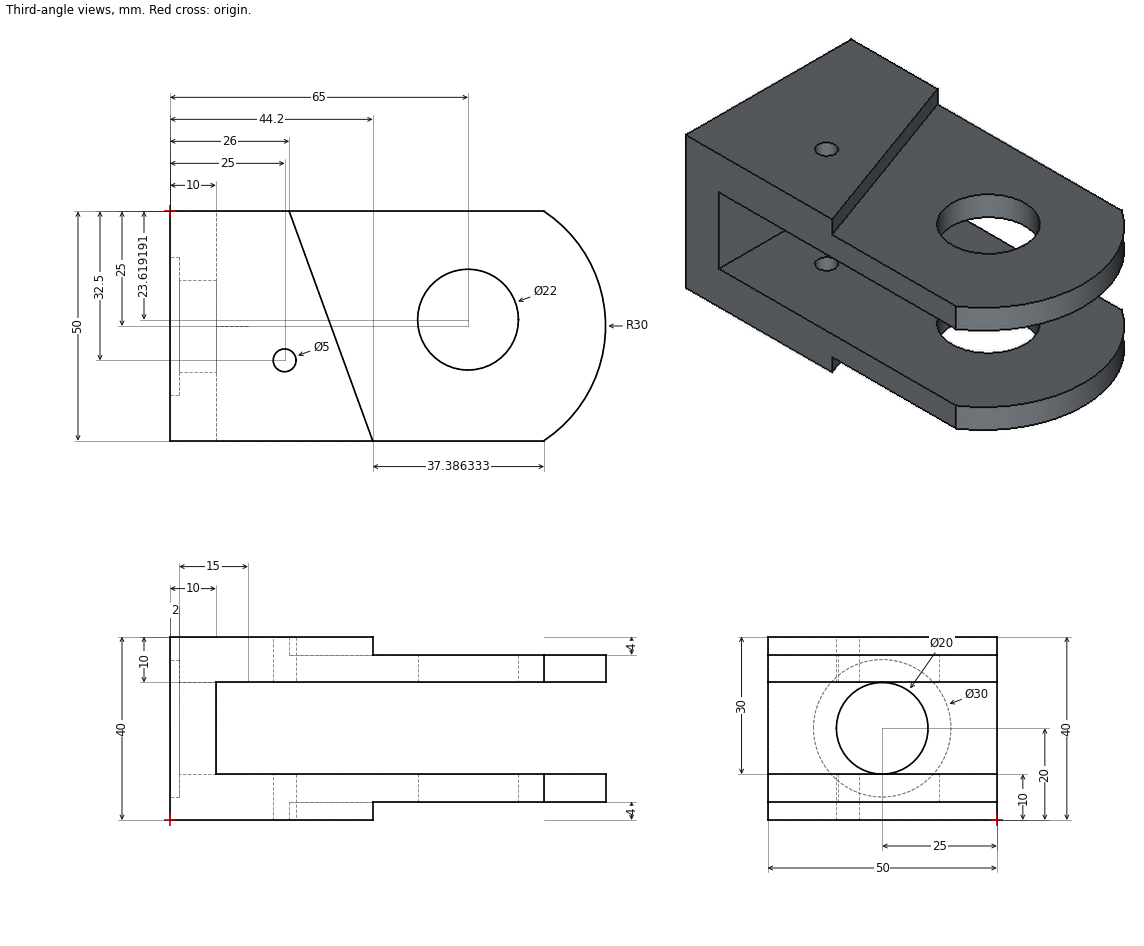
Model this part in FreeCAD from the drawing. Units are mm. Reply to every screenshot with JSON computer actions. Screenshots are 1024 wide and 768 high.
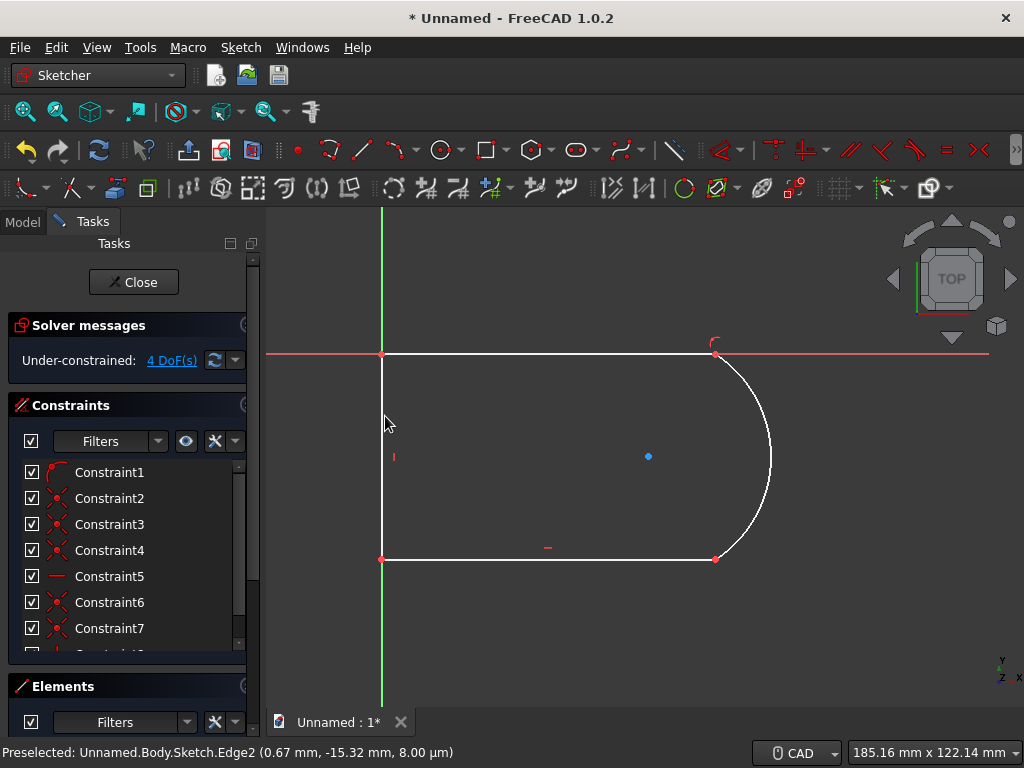
{"action": "left_click", "coordinate": [762, 504]}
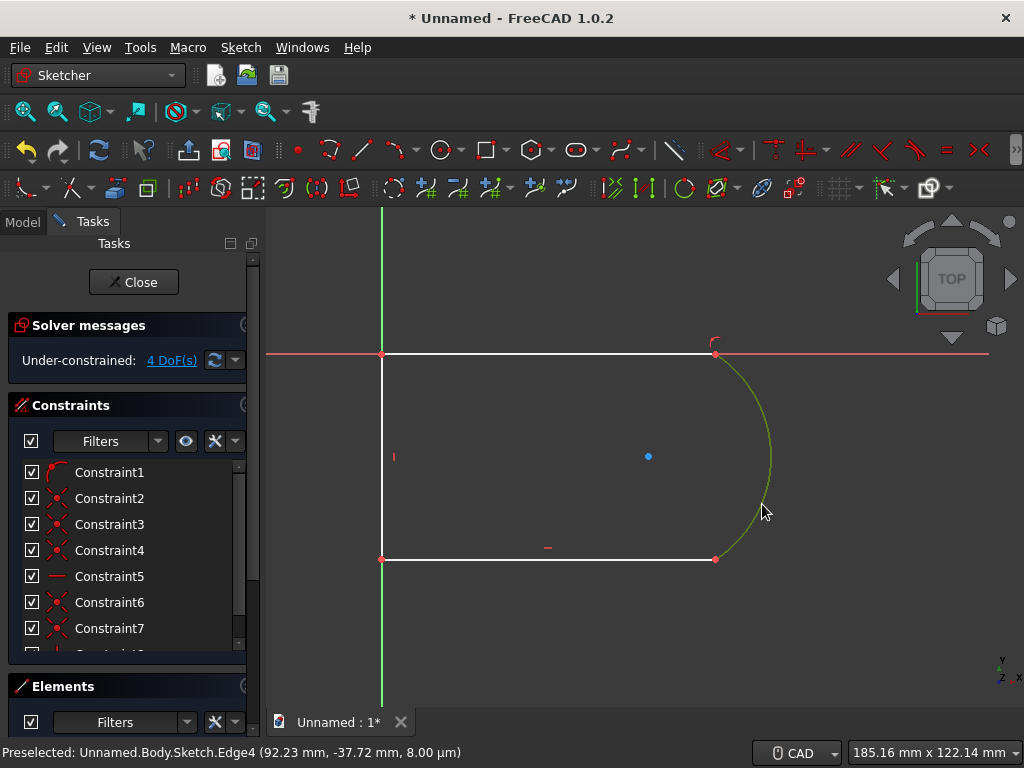
{"action": "key", "text": "k r"}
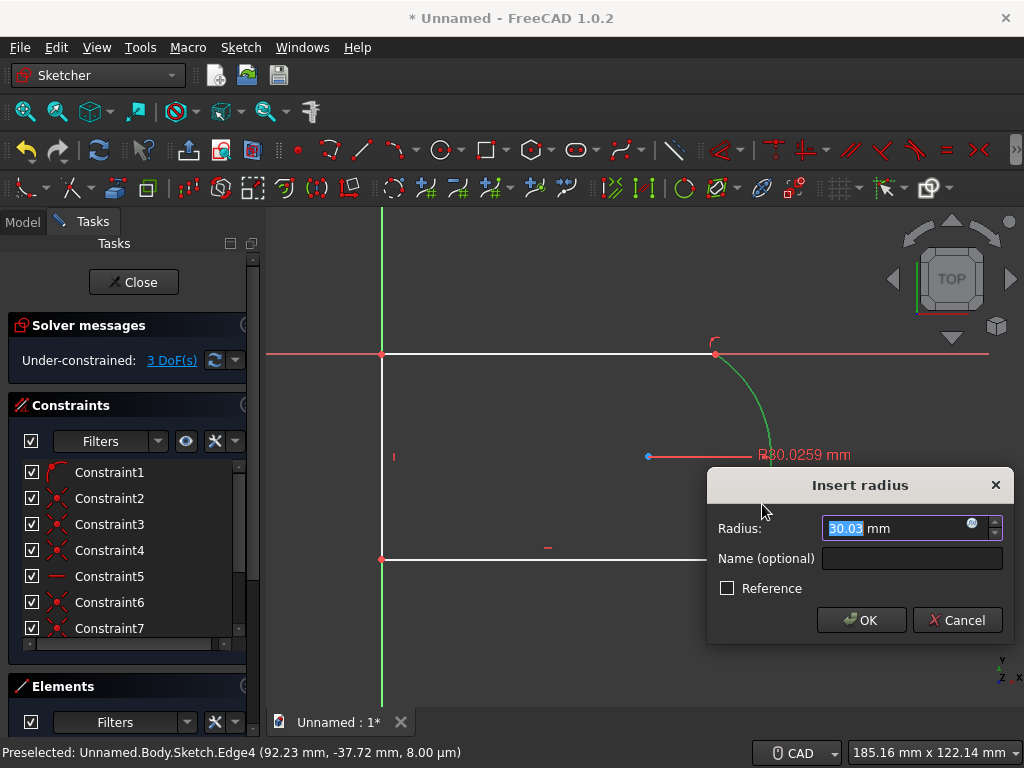
{"action": "type", "text": "30"}
{"action": "key", "text": "Return"}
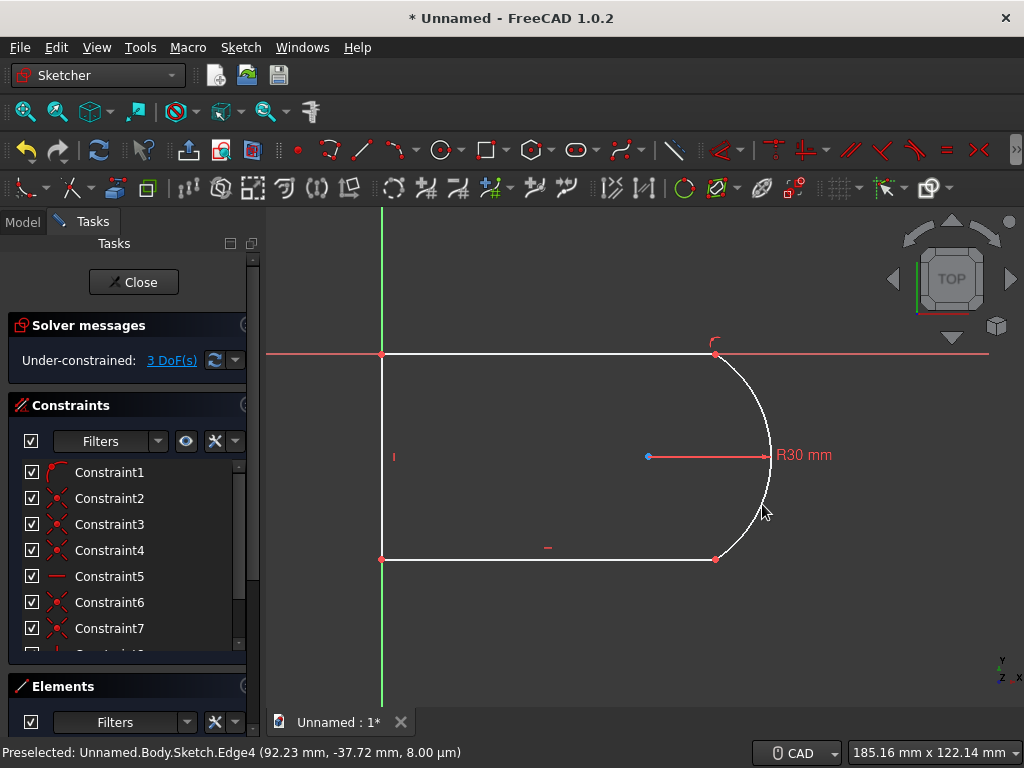
{"action": "left_click", "coordinate": [382, 416]}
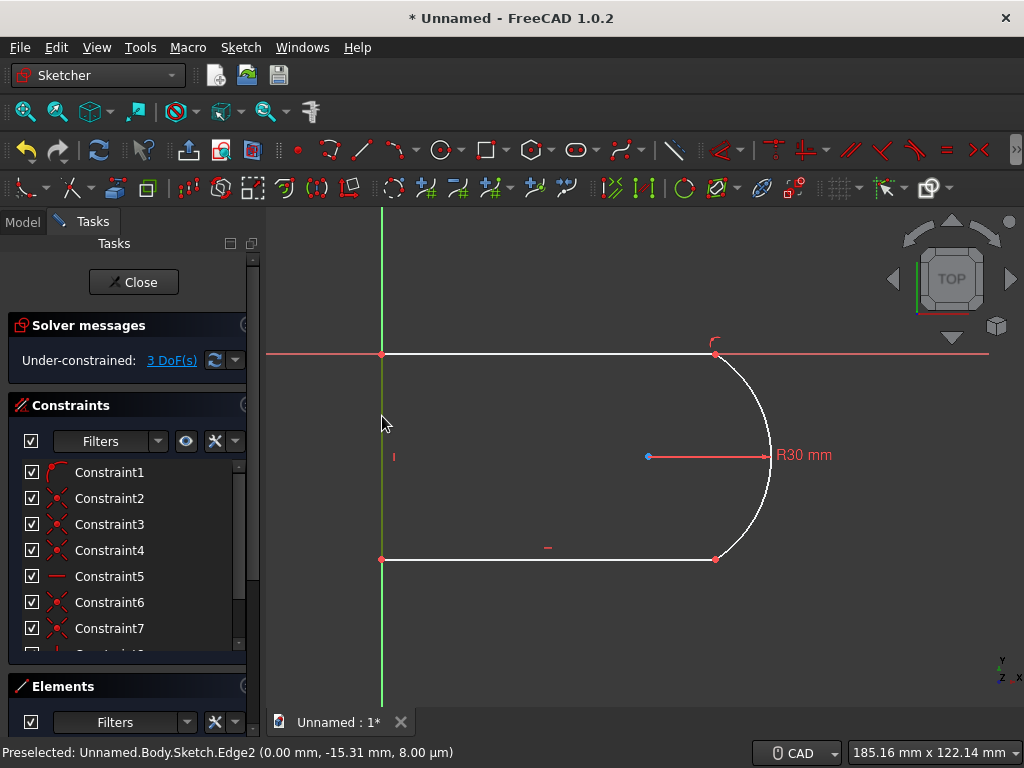
{"action": "left_click", "coordinate": [742, 150]}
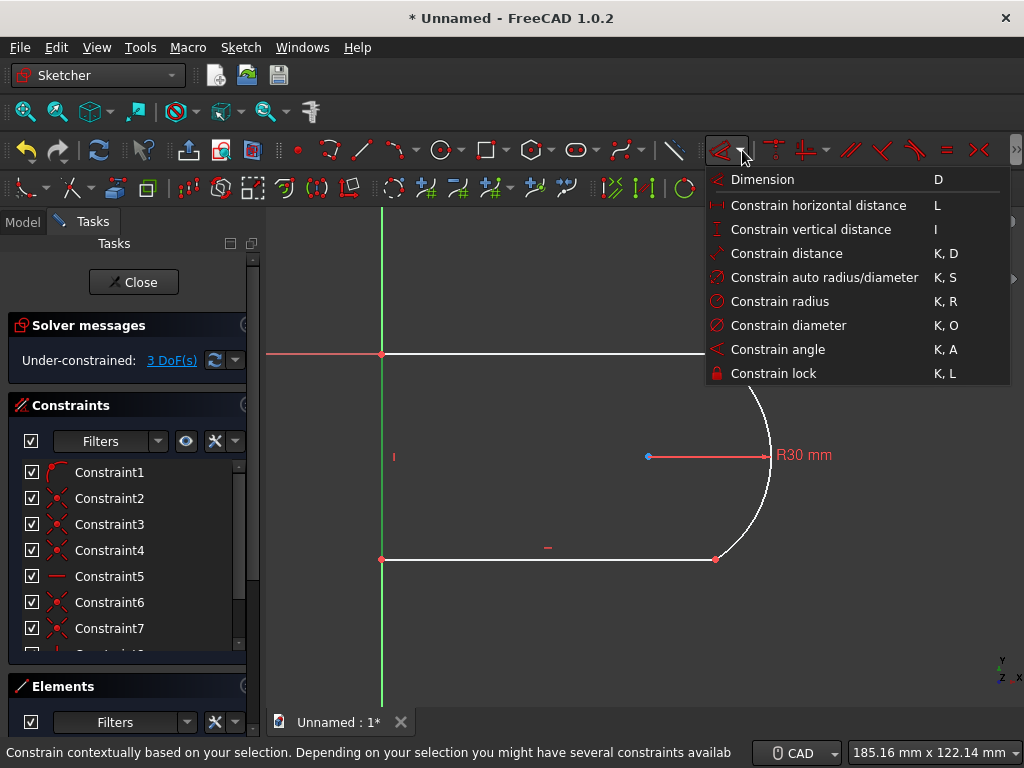
{"action": "left_click", "coordinate": [858, 229]}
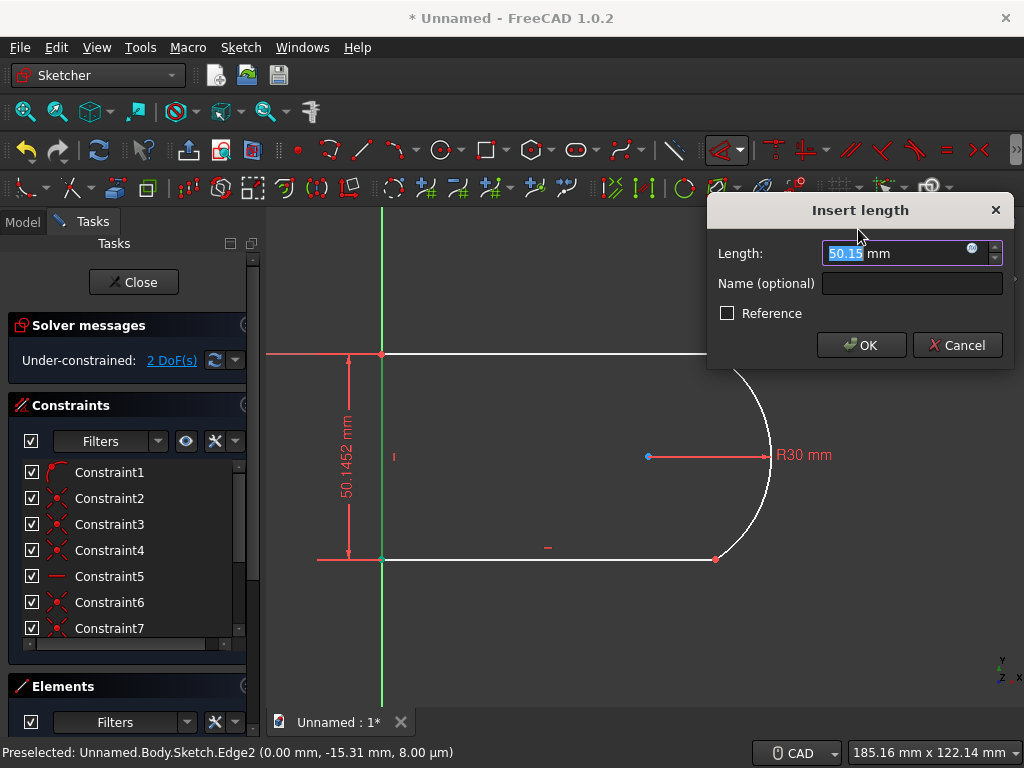
{"action": "type", "text": "50"}
{"action": "key", "text": "Return"}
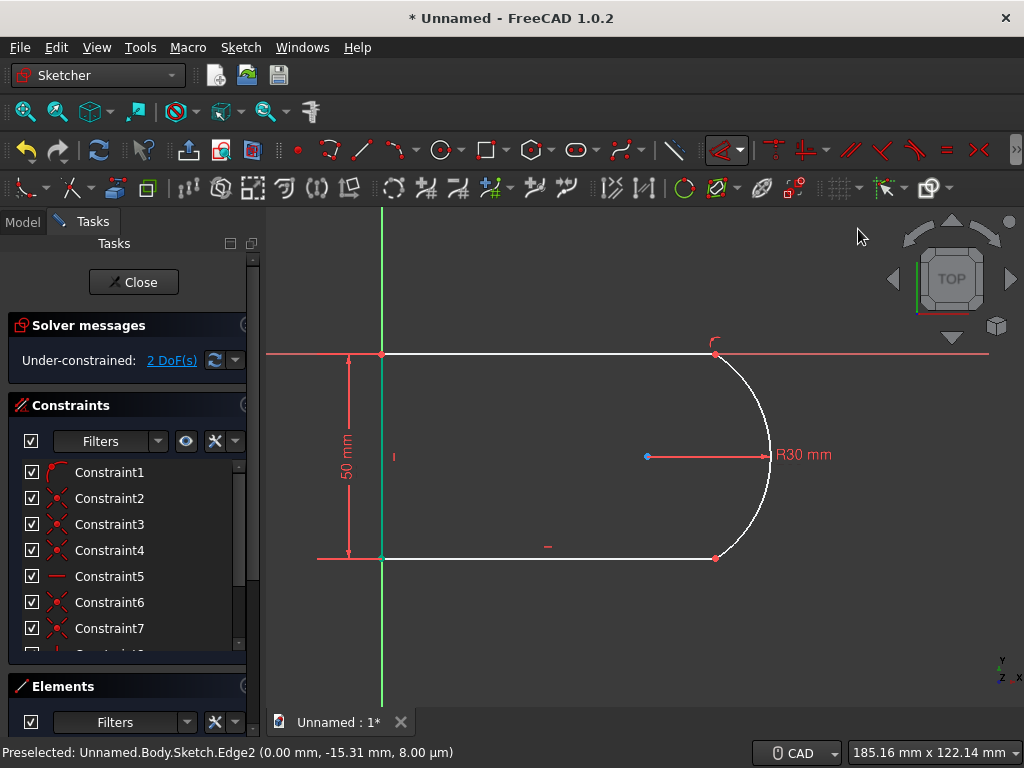
{"action": "left_click", "coordinate": [648, 457]}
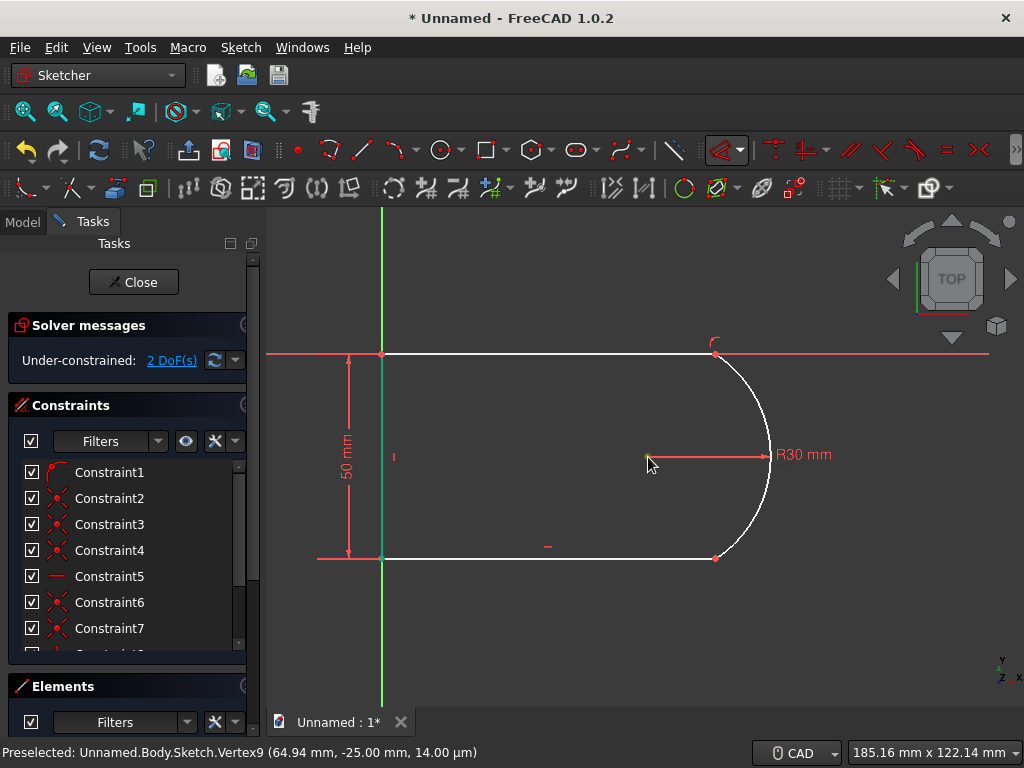
{"action": "key", "text": "l"}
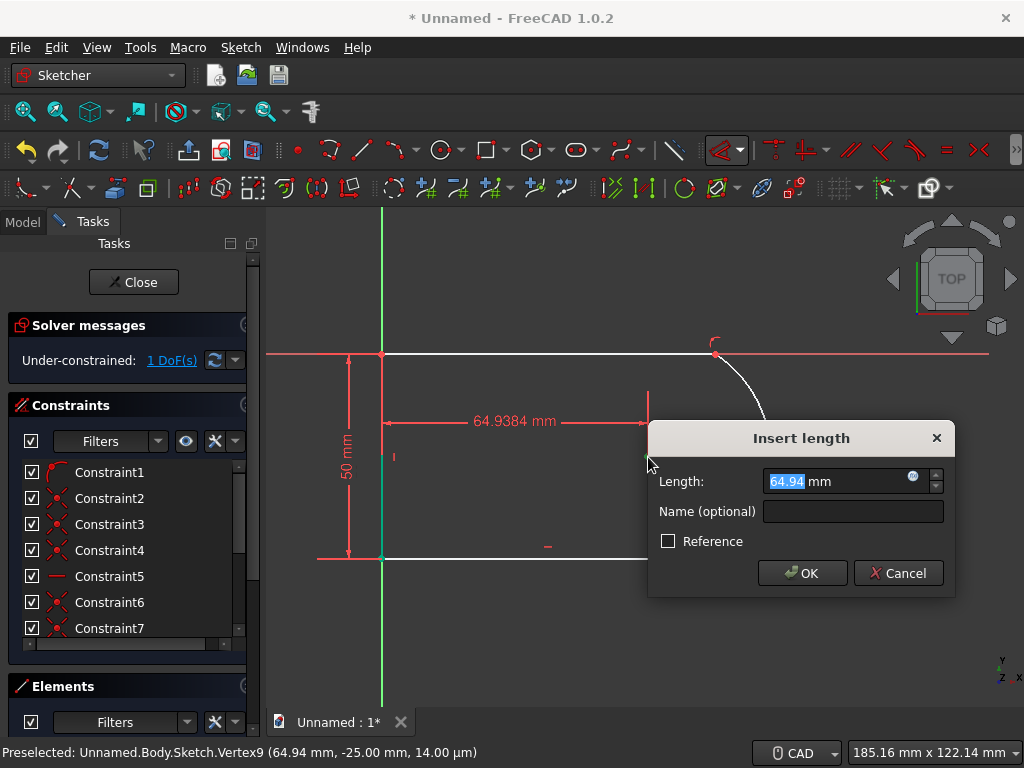
{"action": "type", "text": "65"}
{"action": "key", "text": "Return"}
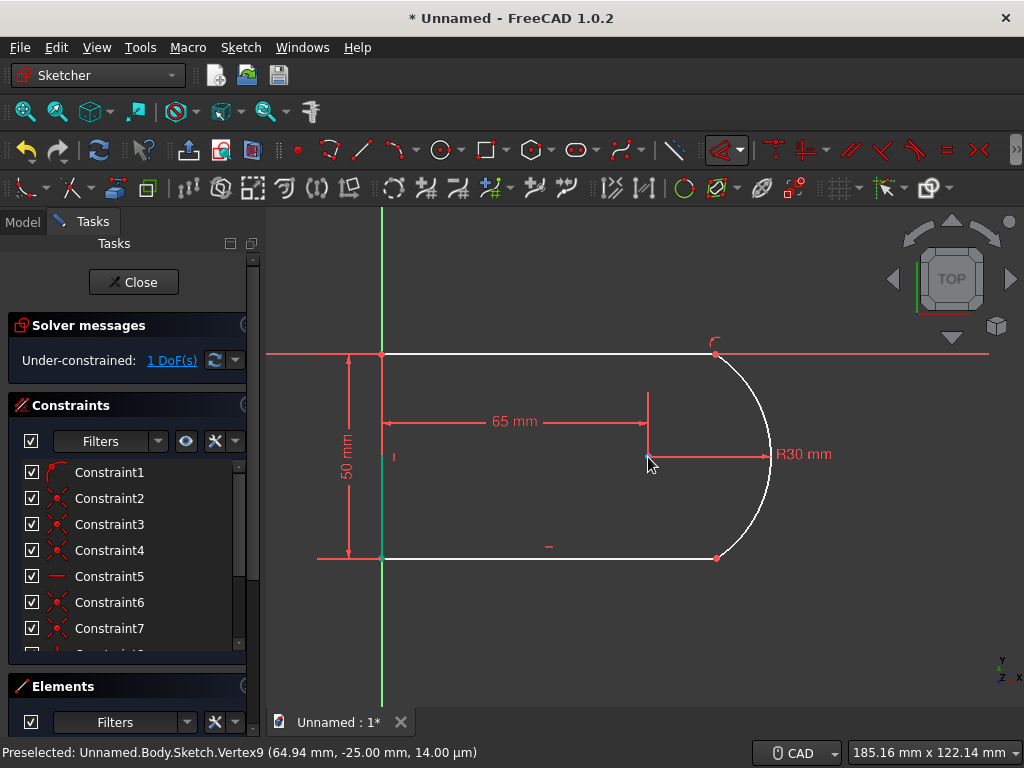
{"action": "left_click", "coordinate": [648, 457]}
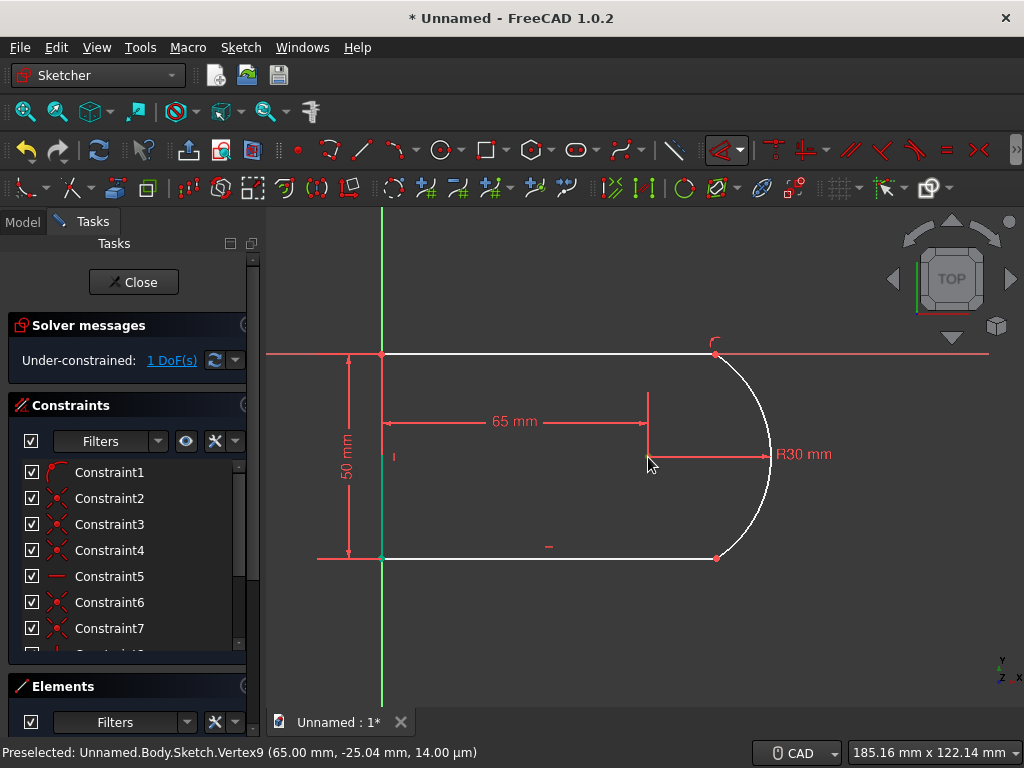
{"action": "left_click", "coordinate": [742, 150]}